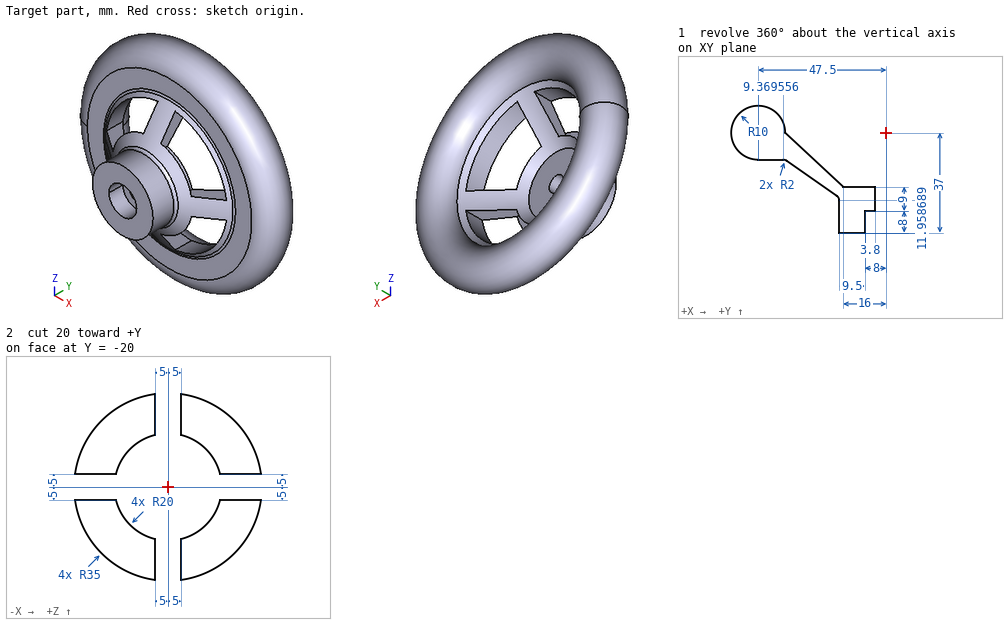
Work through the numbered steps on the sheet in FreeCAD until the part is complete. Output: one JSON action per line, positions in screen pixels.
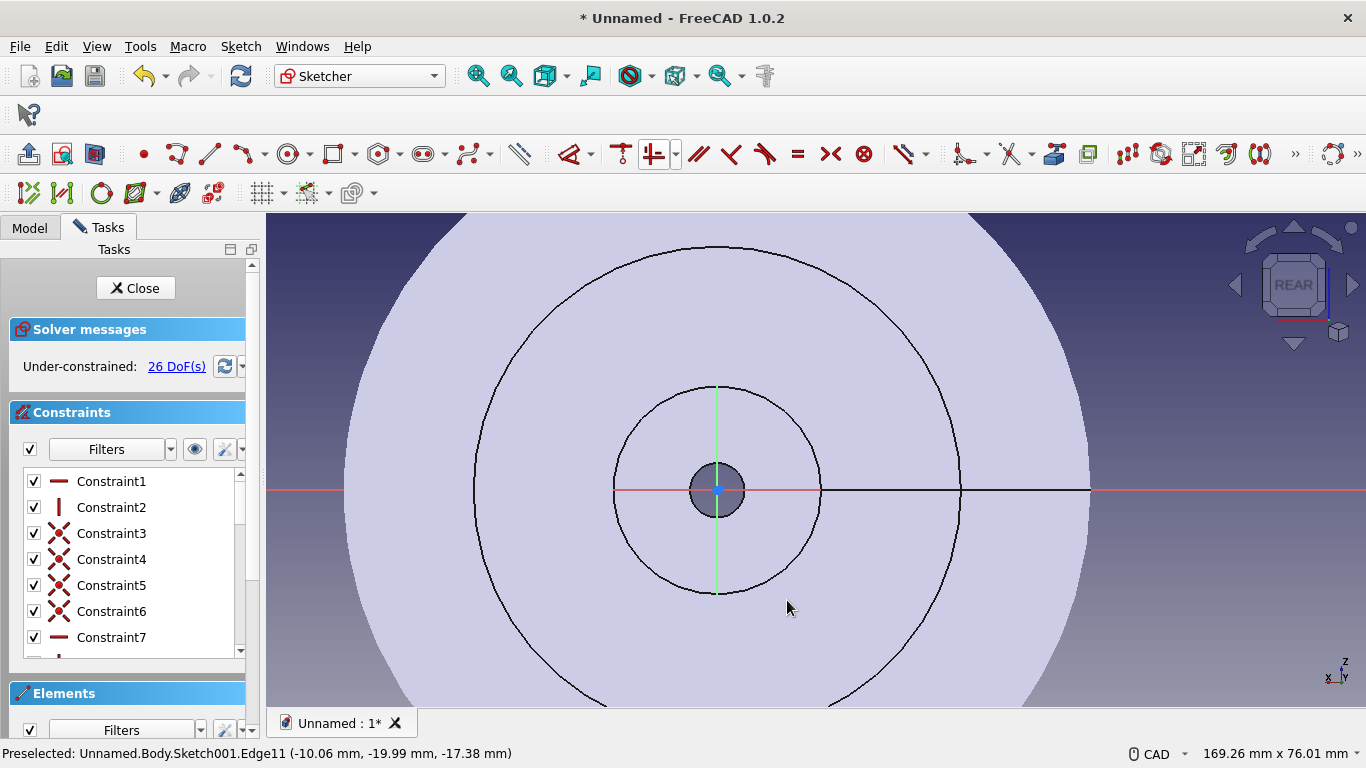
{"action": "key", "text": "c"}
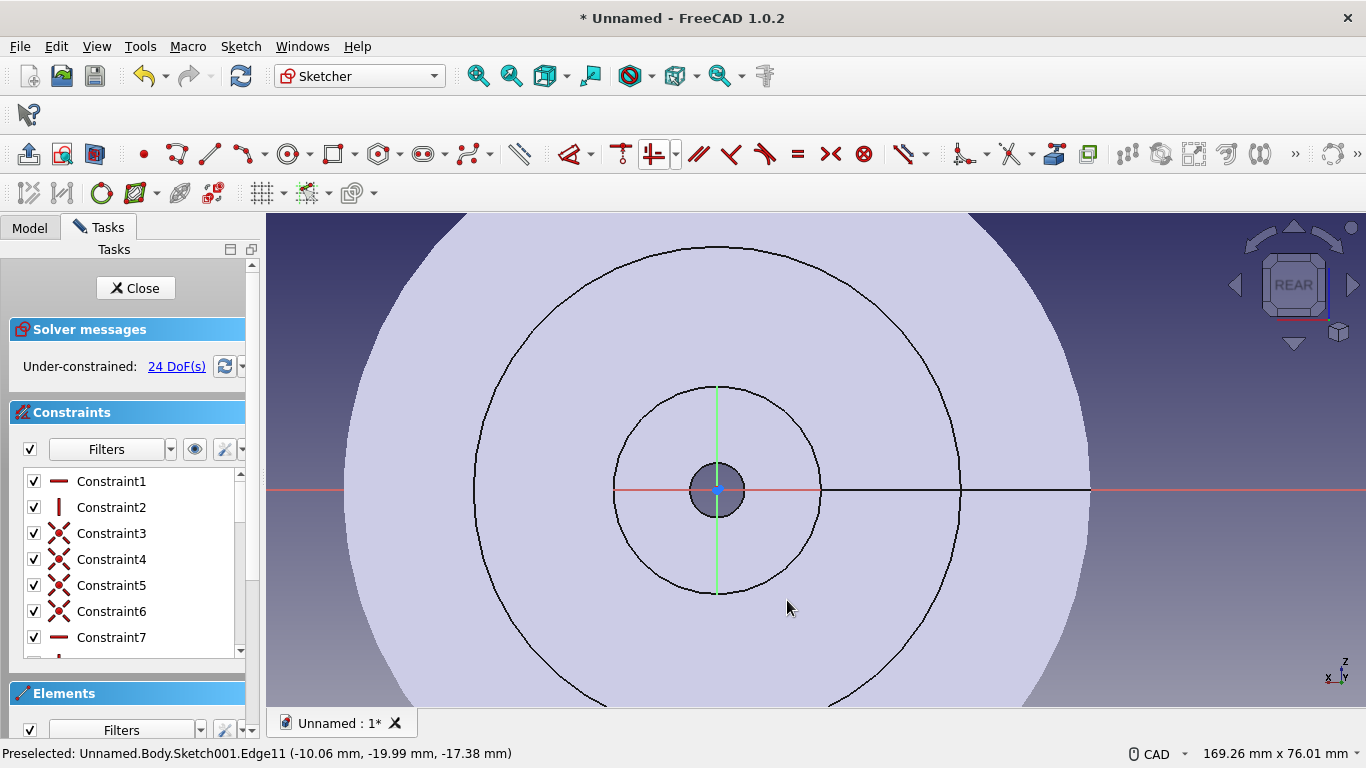
{"action": "left_click", "coordinate": [521, 606]}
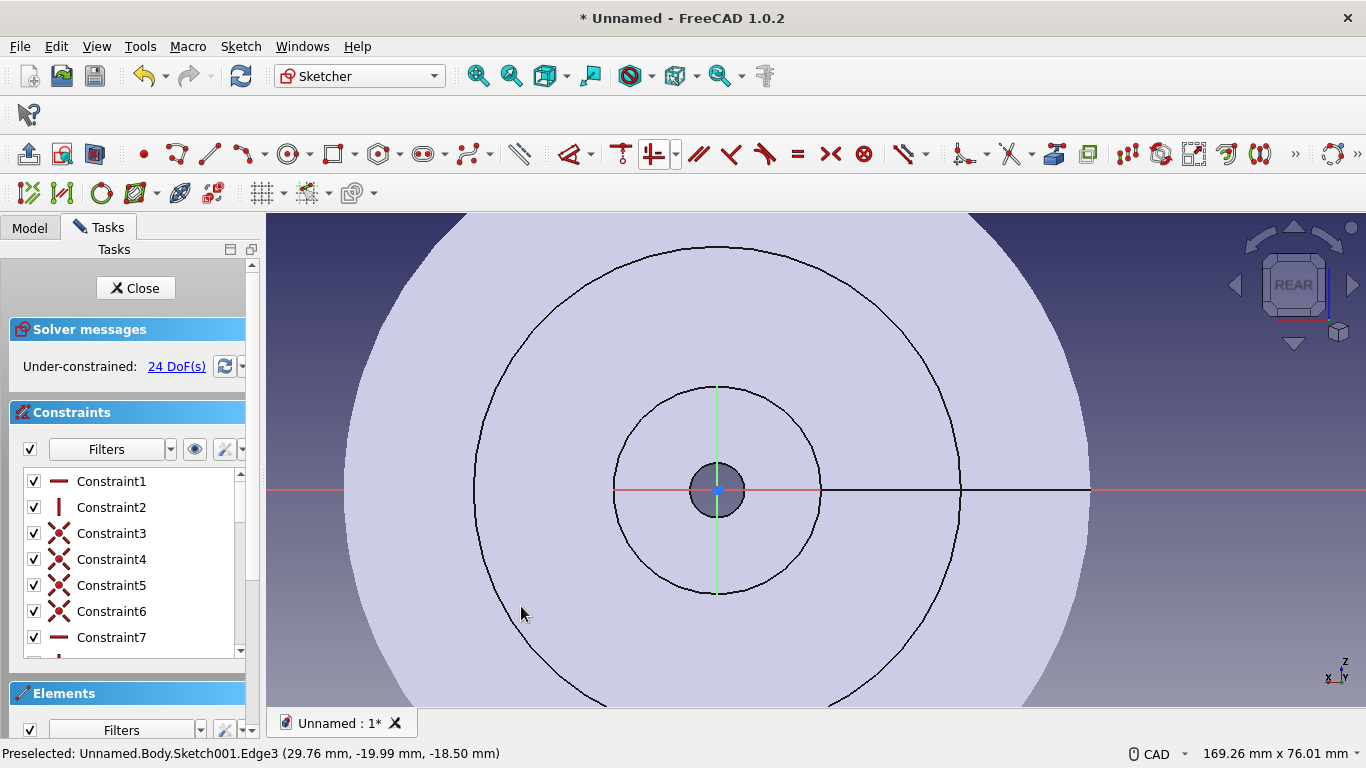
{"action": "left_click", "coordinate": [913, 606]}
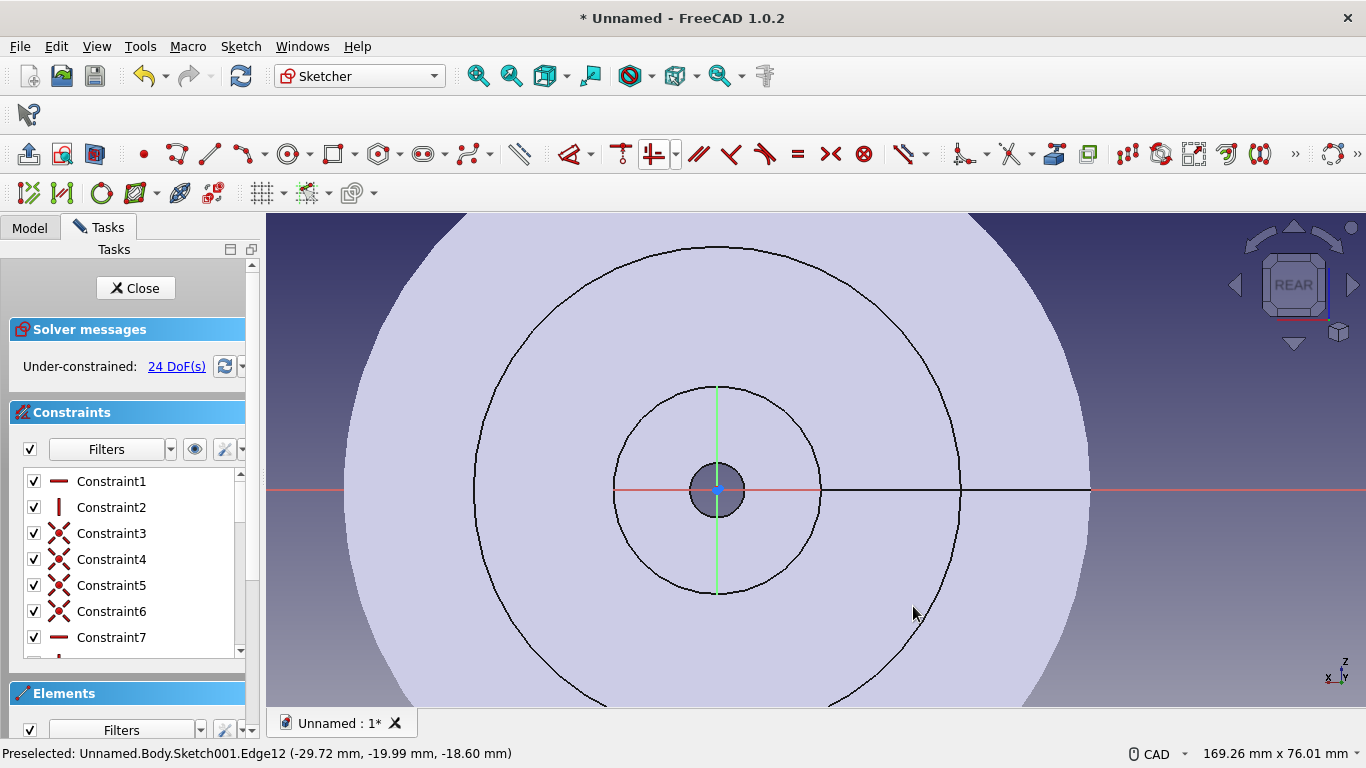
{"action": "key", "text": "c"}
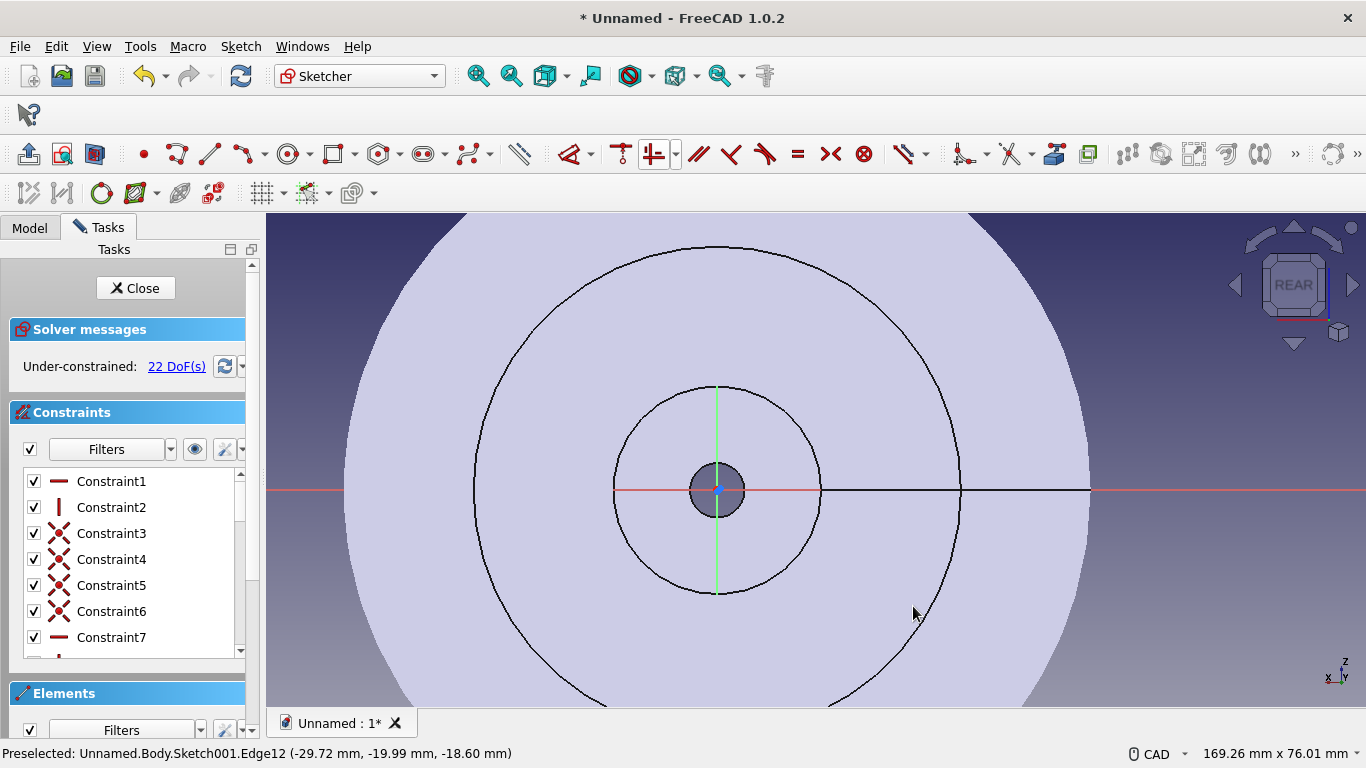
{"action": "left_click", "coordinate": [521, 606]}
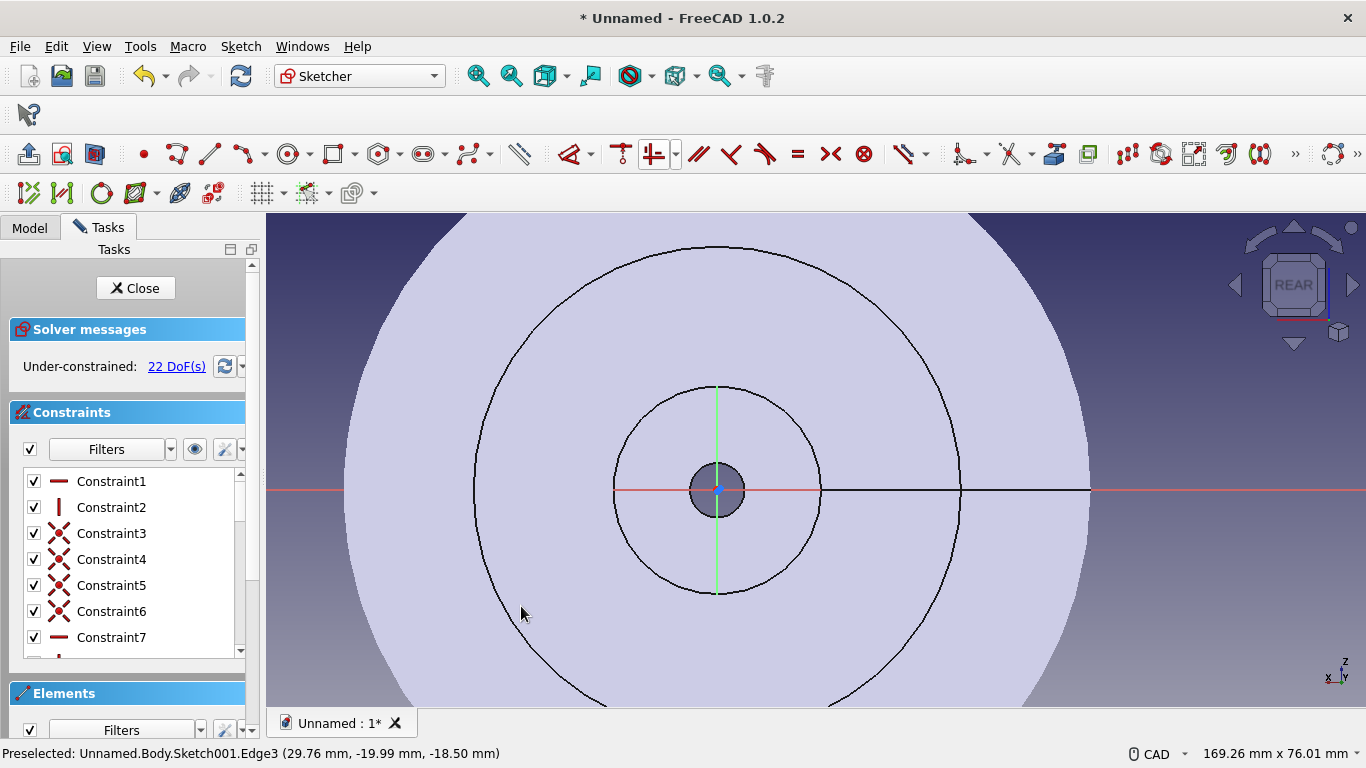
{"action": "left_click", "coordinate": [827, 421]}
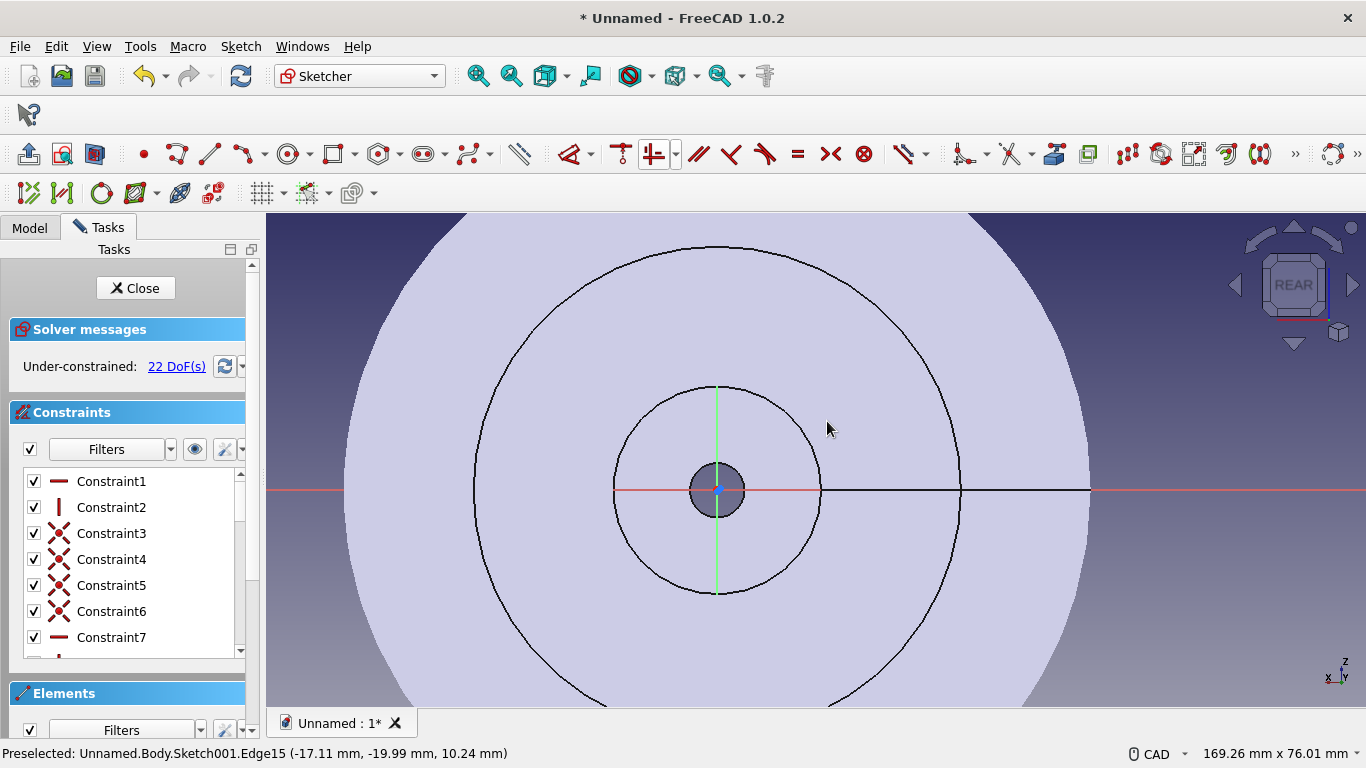
{"action": "key", "text": "c"}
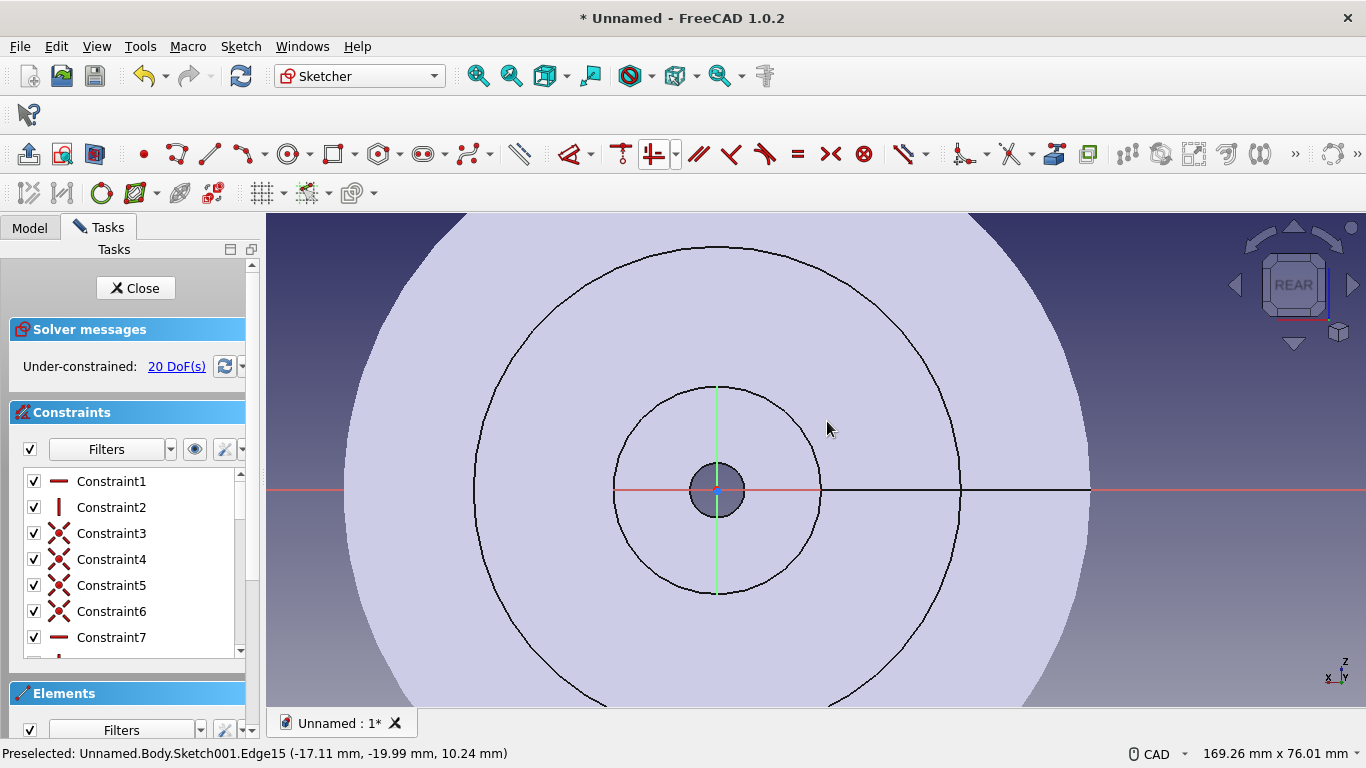
{"action": "left_click", "coordinate": [521, 606]}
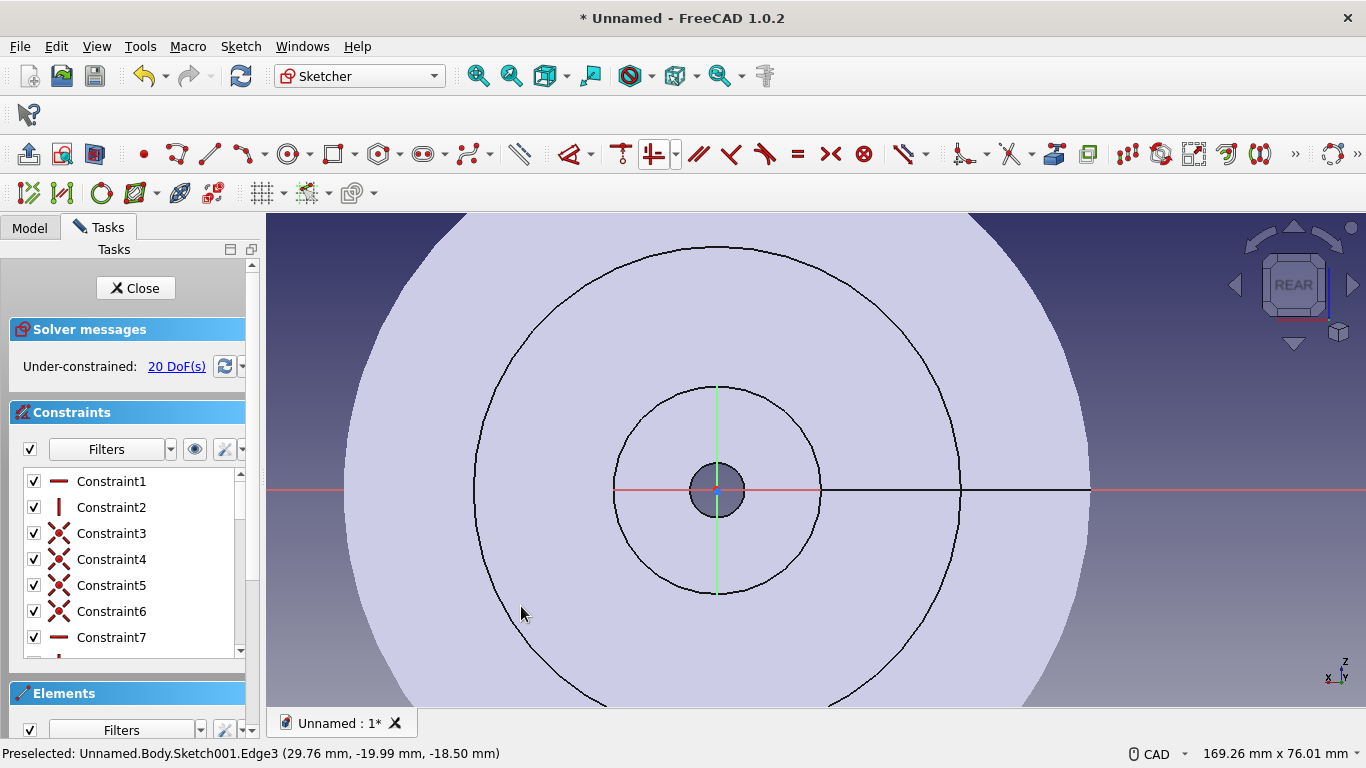
{"action": "left_click", "coordinate": [914, 377]}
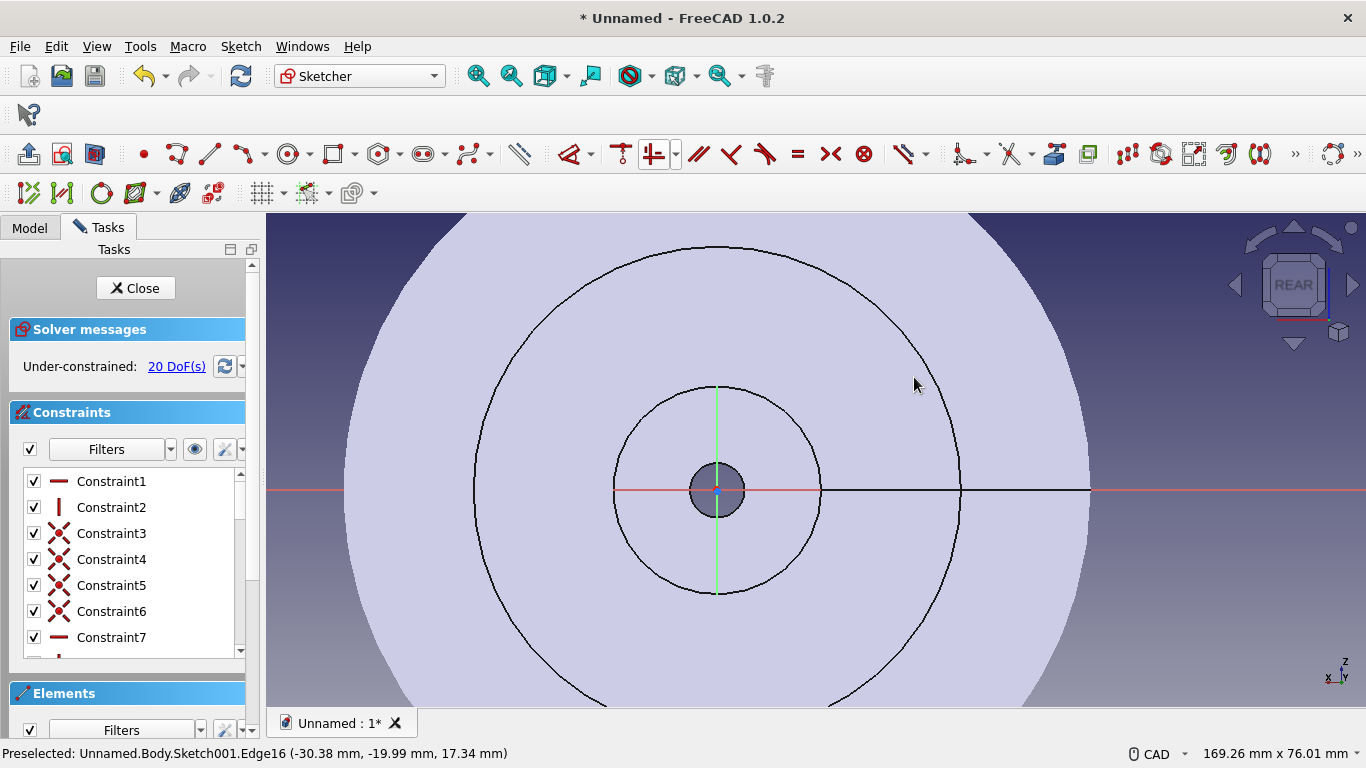
{"action": "left_click", "coordinate": [621, 154]}